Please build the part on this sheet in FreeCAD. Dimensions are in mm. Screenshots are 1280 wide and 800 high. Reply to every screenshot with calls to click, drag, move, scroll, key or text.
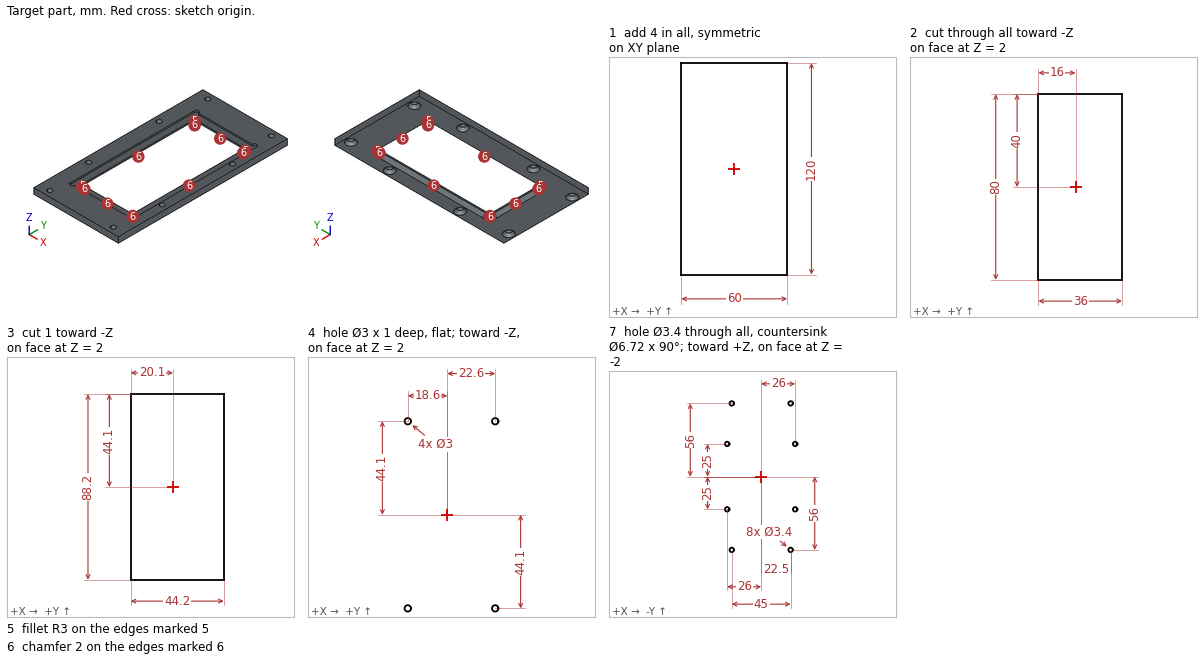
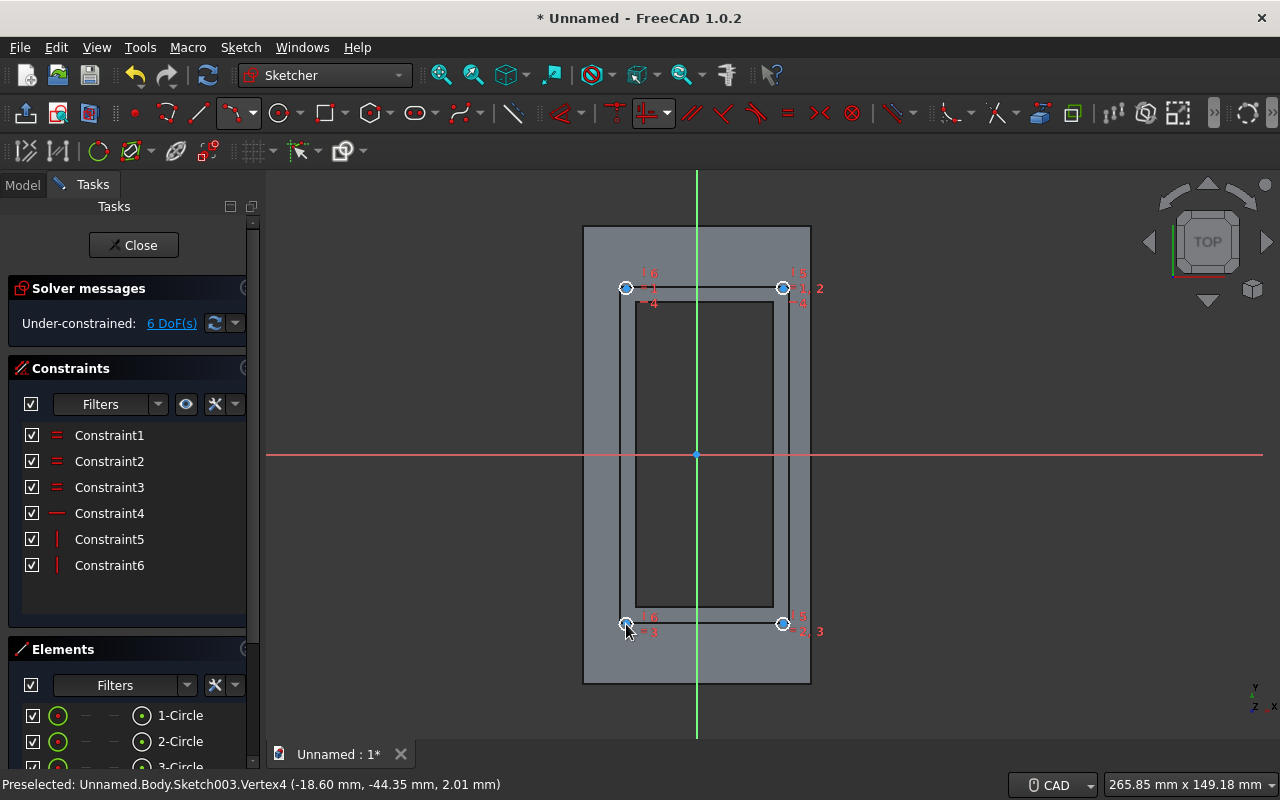
click(783, 624)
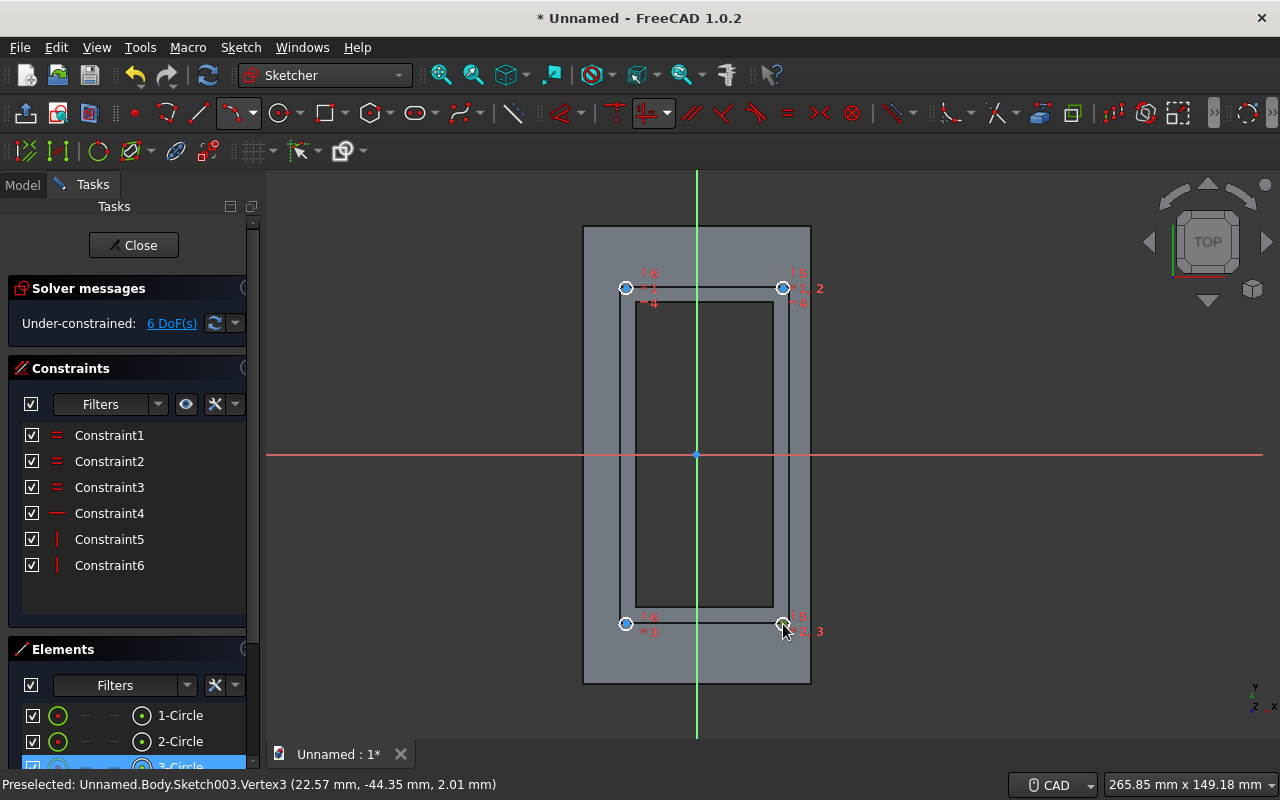
click(626, 624)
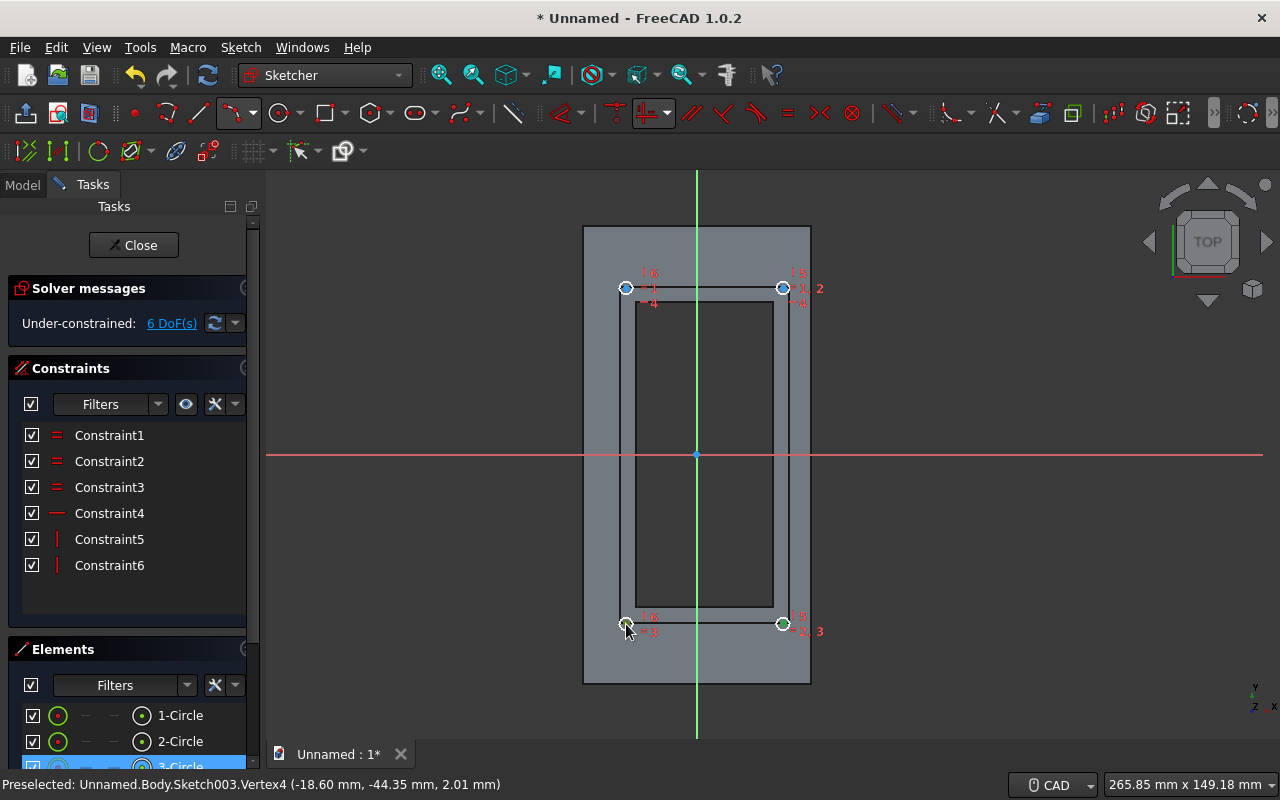
click(670, 114)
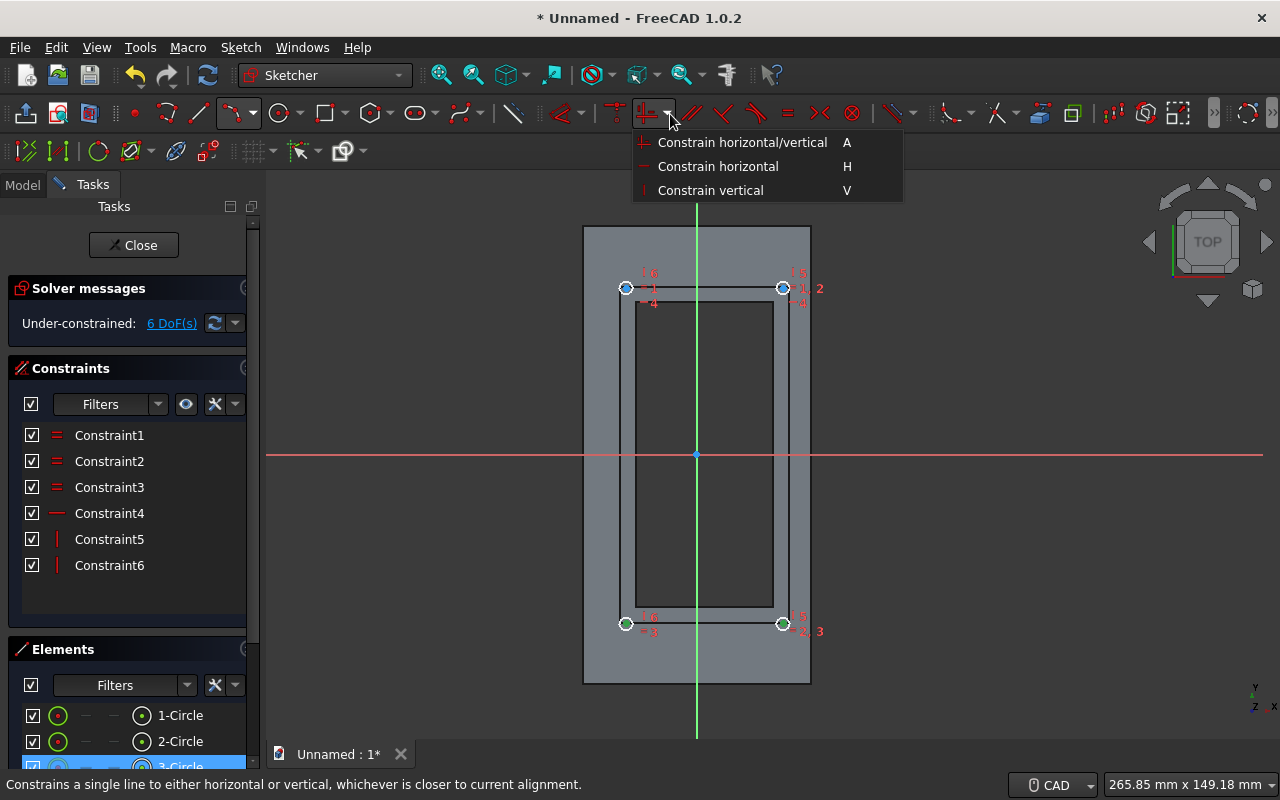
click(768, 166)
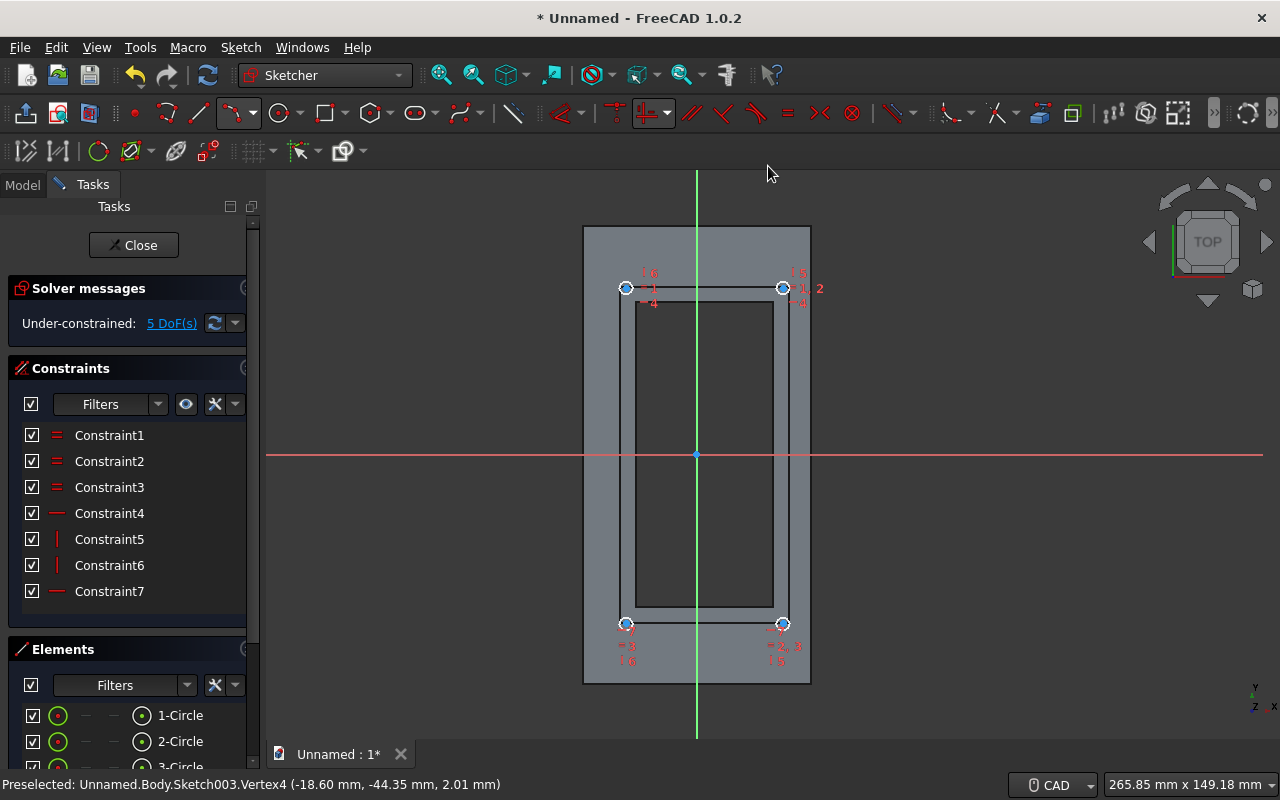
click(560, 114)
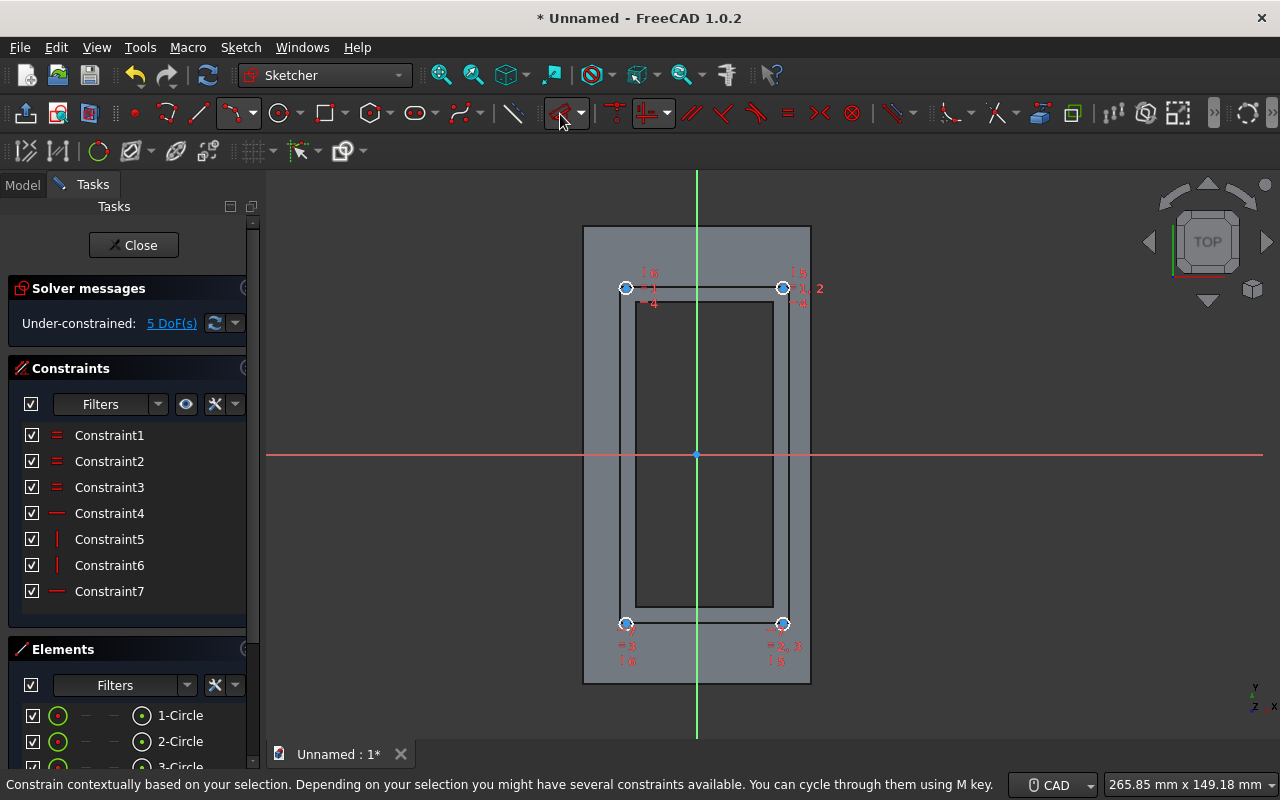
scroll(631, 283, up, 7)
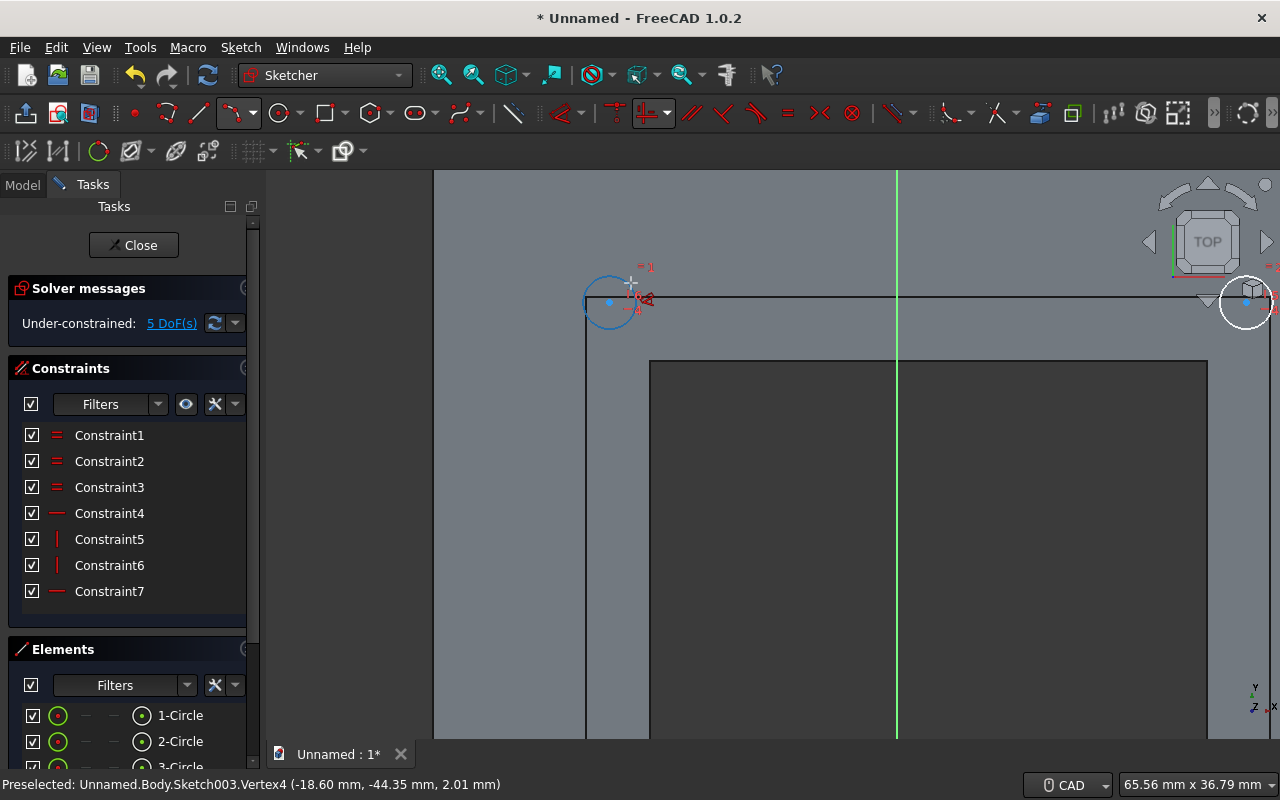
click(628, 284)
click(650, 261)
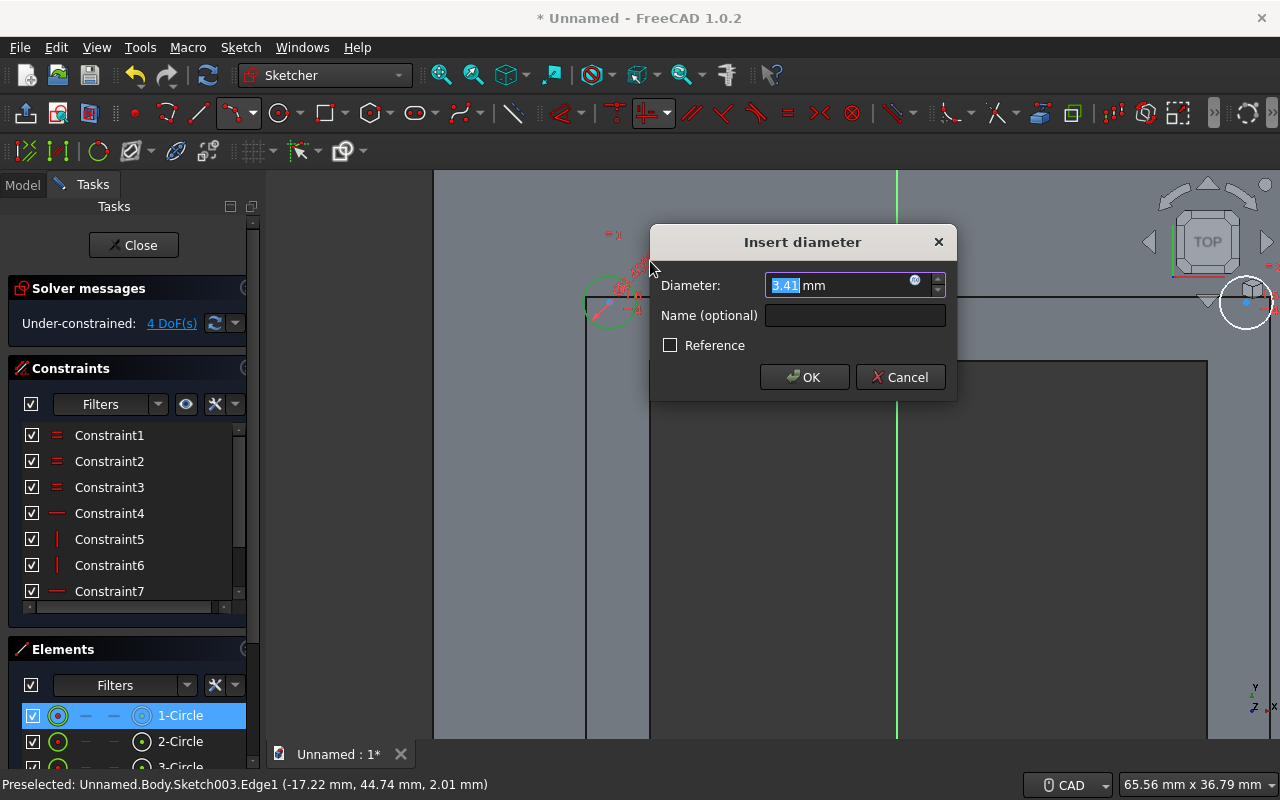
text(3)
key(Return)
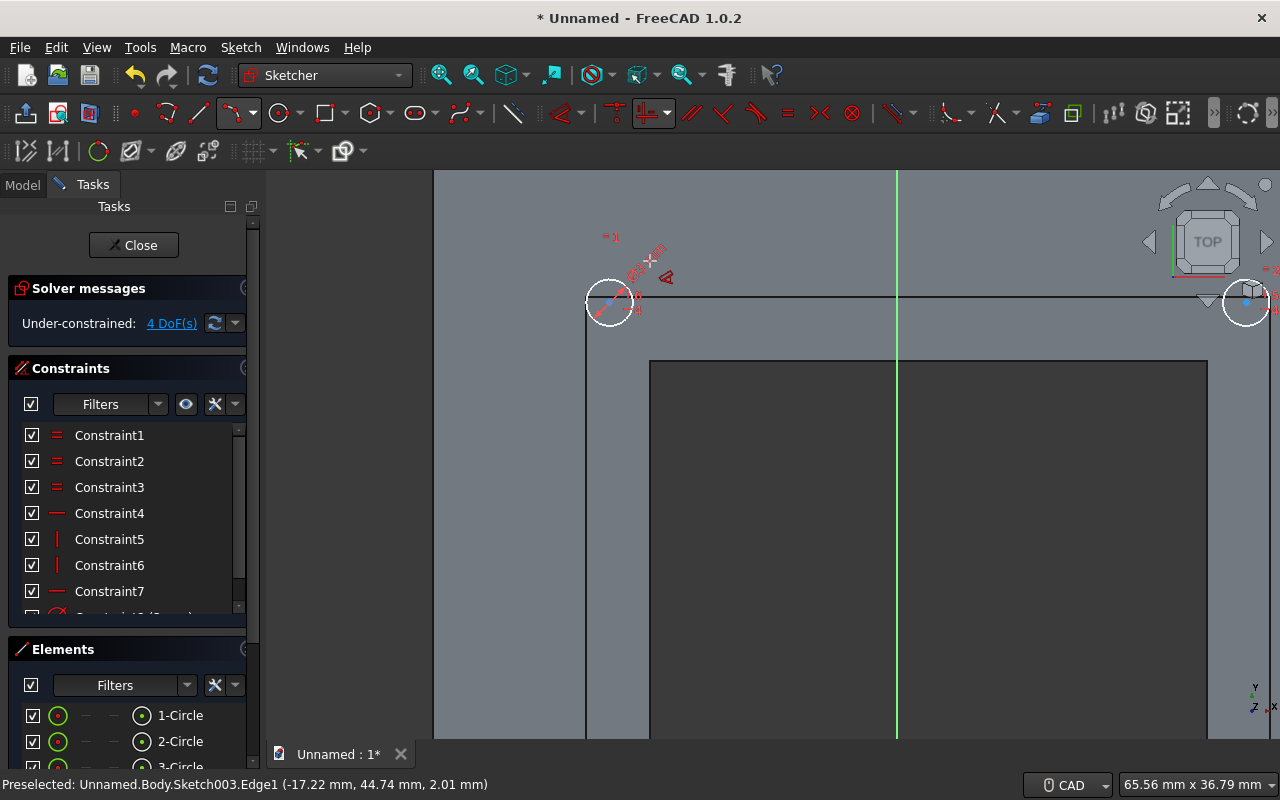
scroll(631, 283, down, 7)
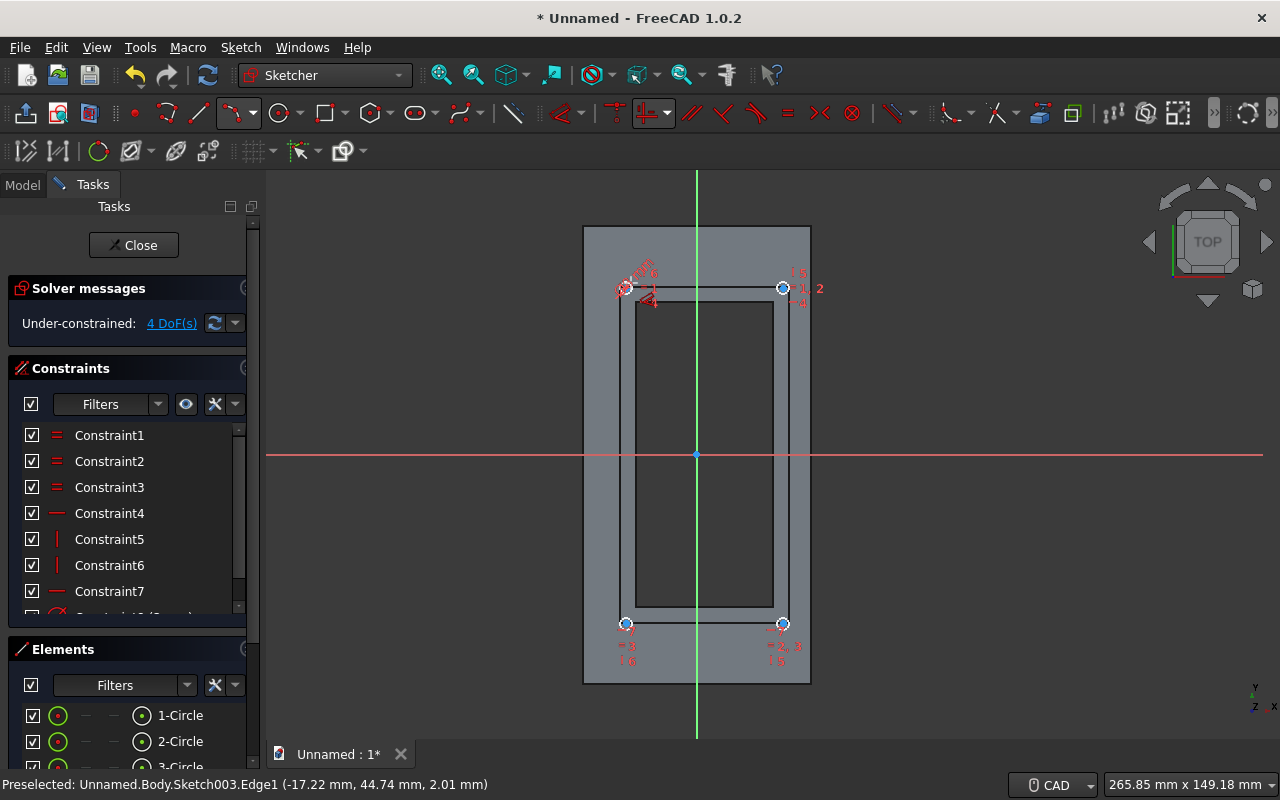
click(626, 288)
click(661, 254)